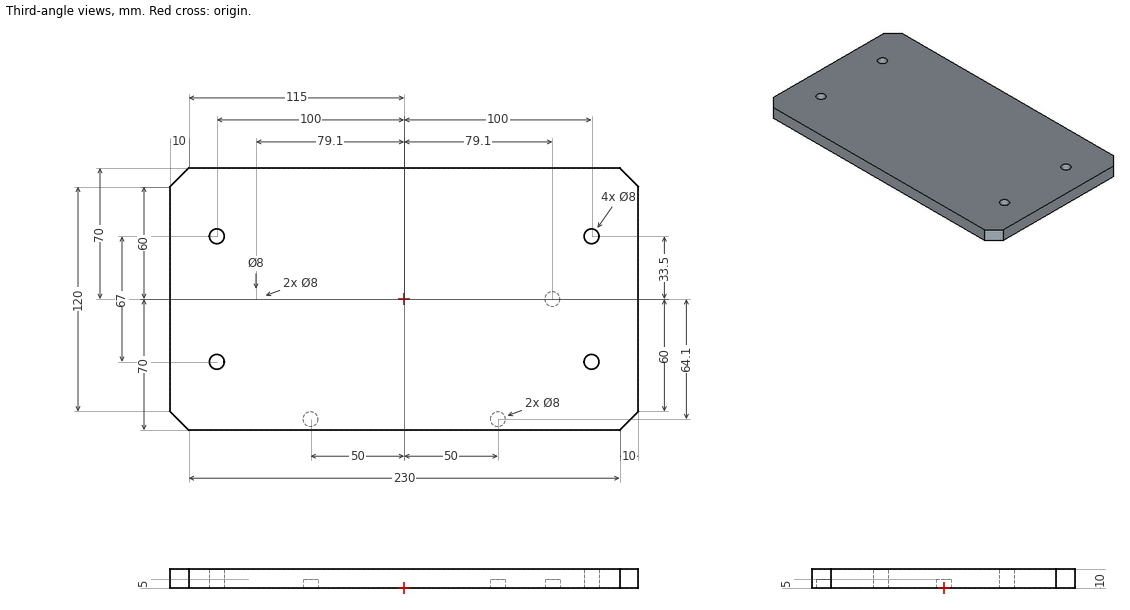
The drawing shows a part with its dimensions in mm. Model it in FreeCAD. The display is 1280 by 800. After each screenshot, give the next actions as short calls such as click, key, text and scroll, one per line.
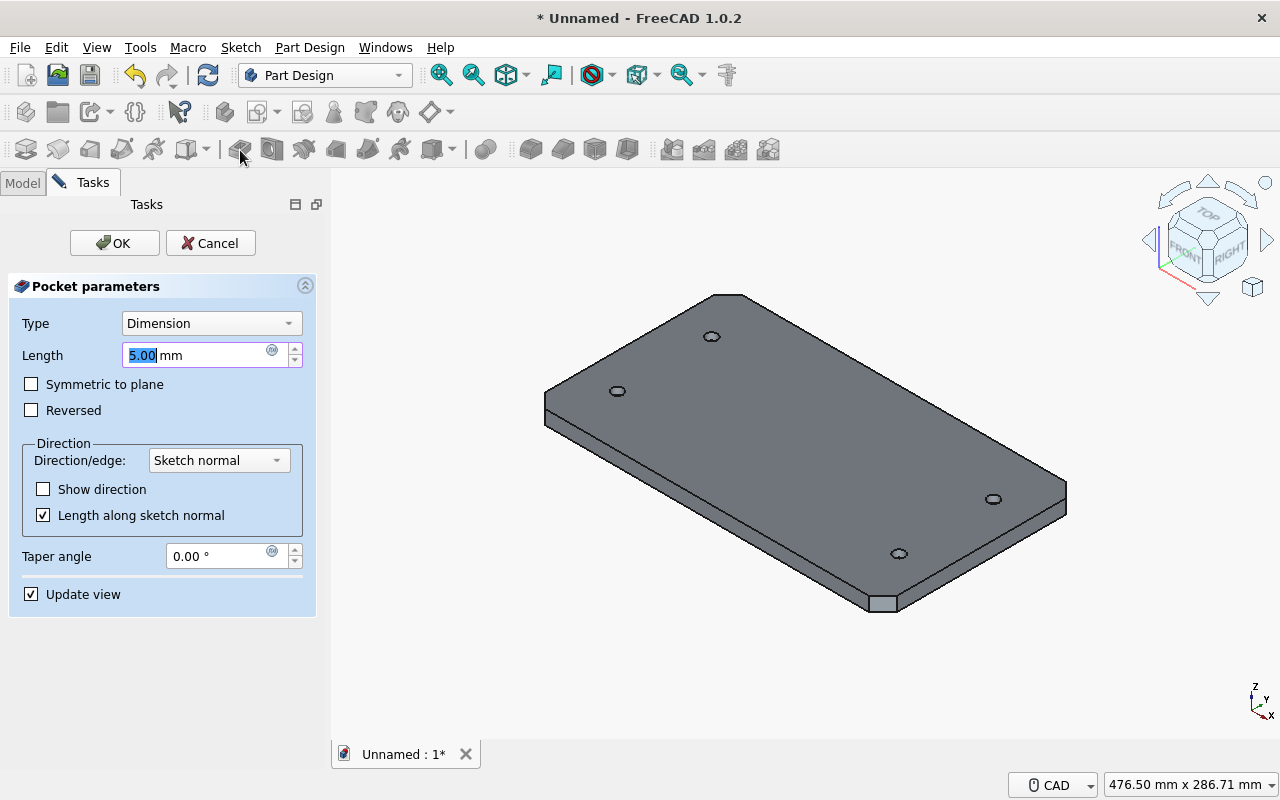
text(10)
key(Tab)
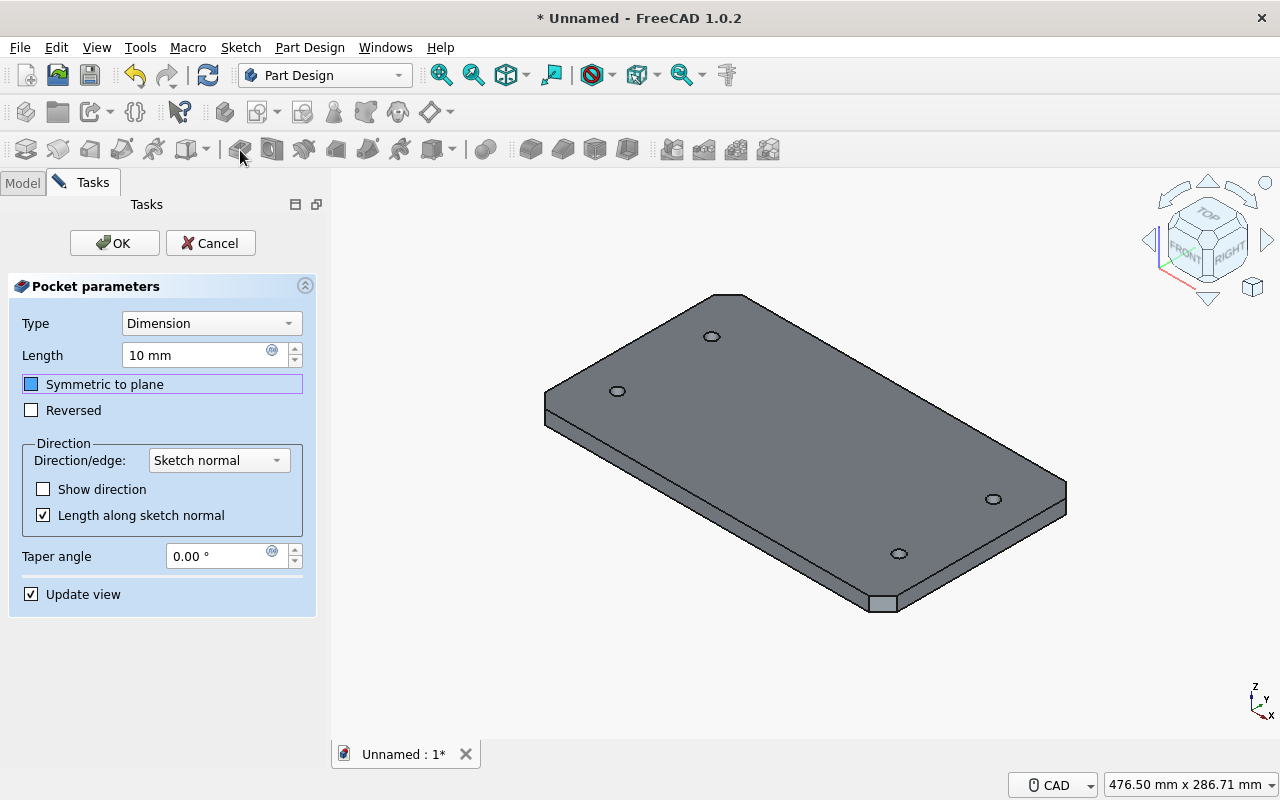
click(115, 243)